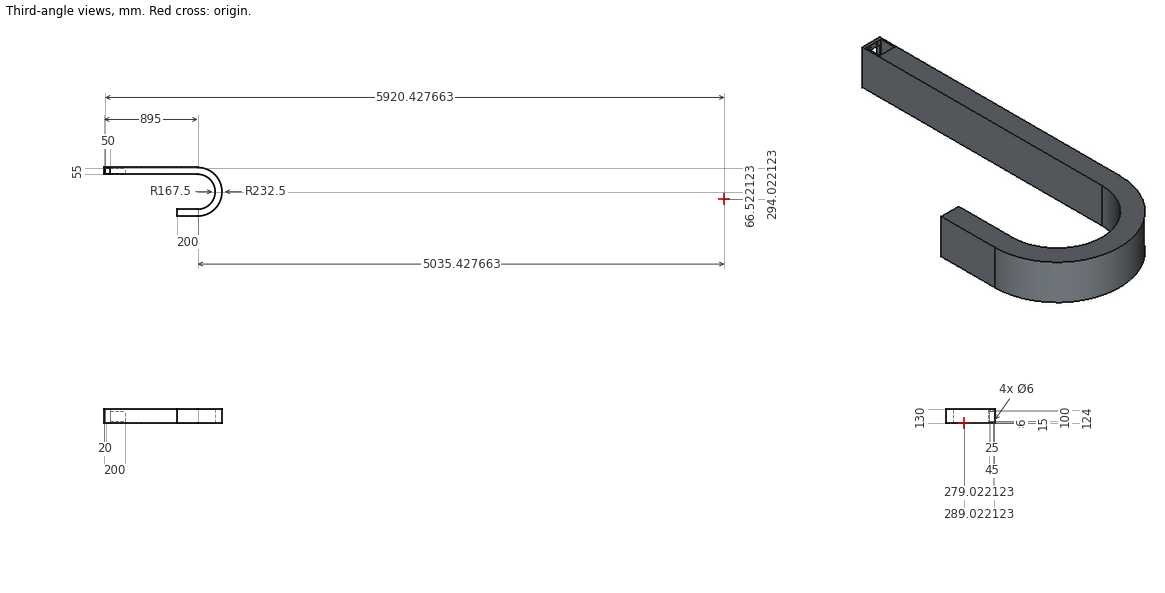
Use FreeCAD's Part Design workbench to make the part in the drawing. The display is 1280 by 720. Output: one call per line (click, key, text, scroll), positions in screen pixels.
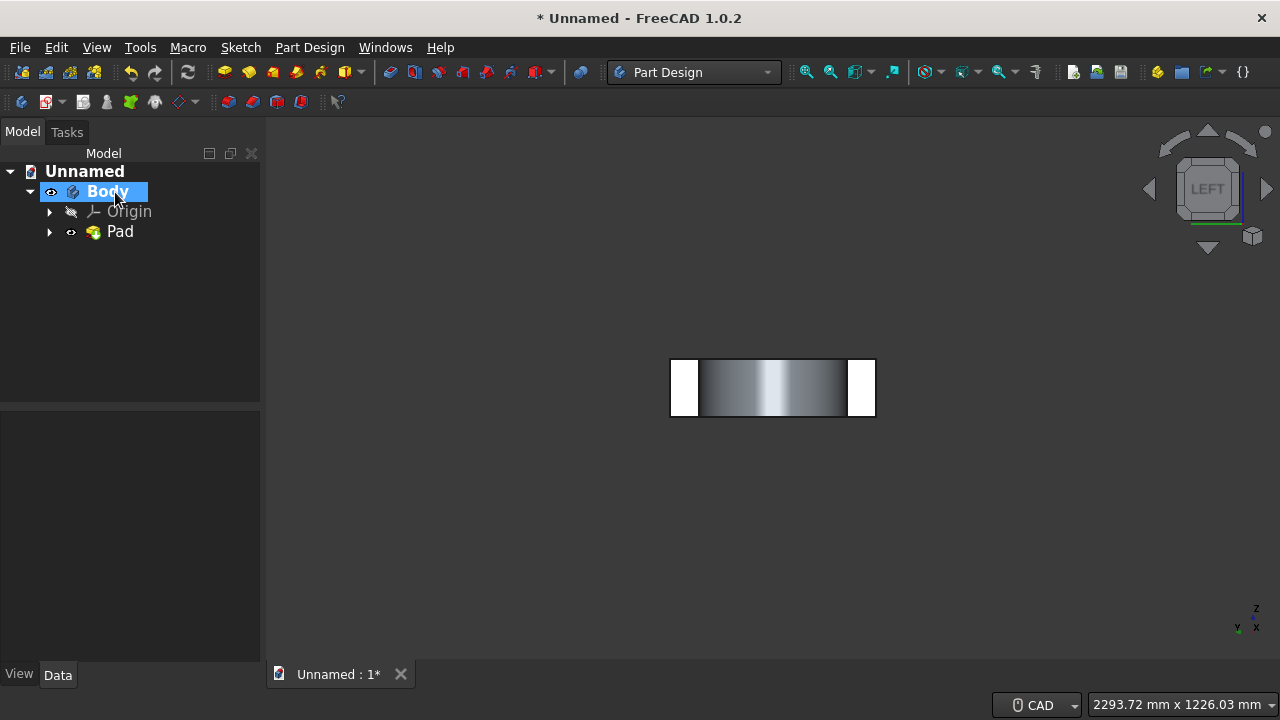
key(v)
key(f)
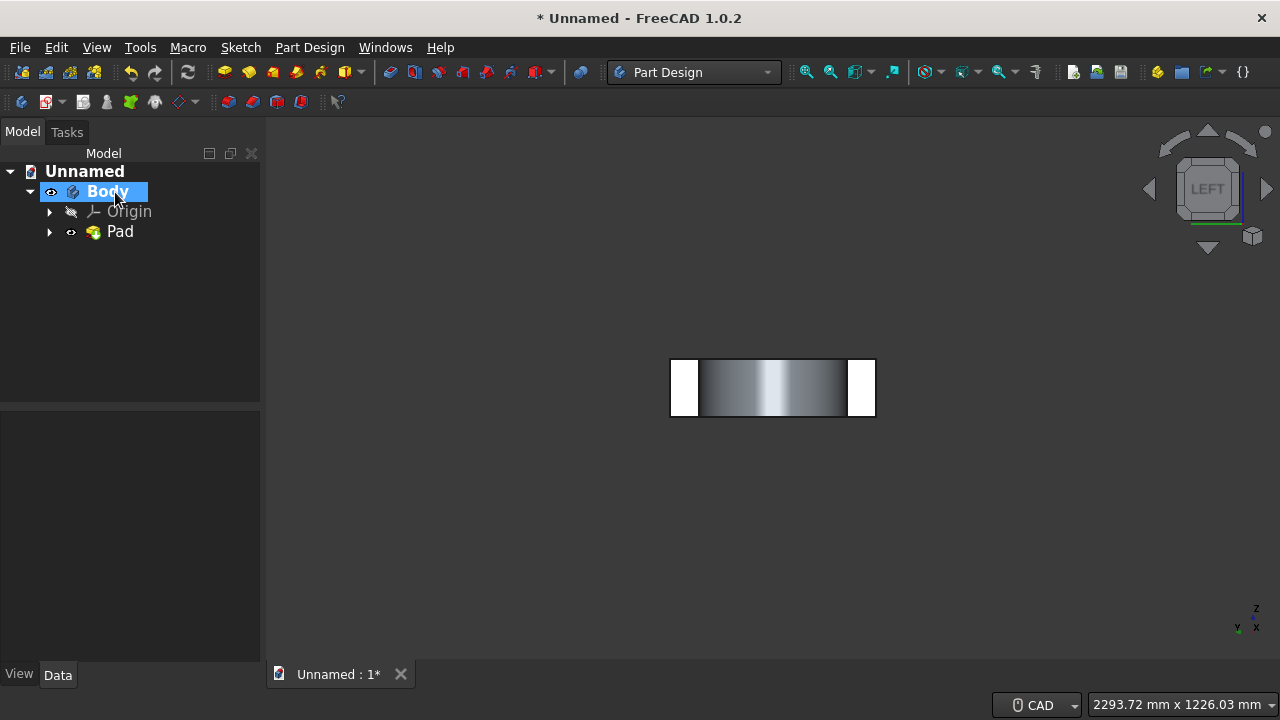
click(685, 379)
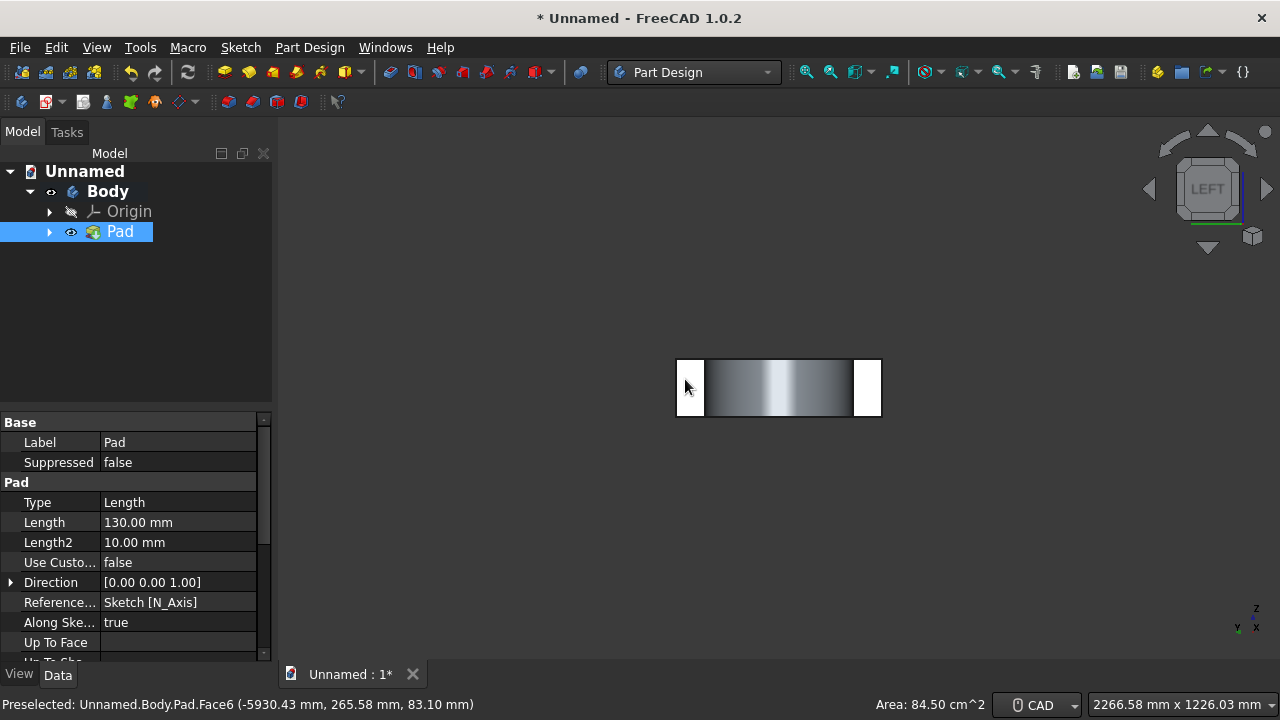
click(46, 102)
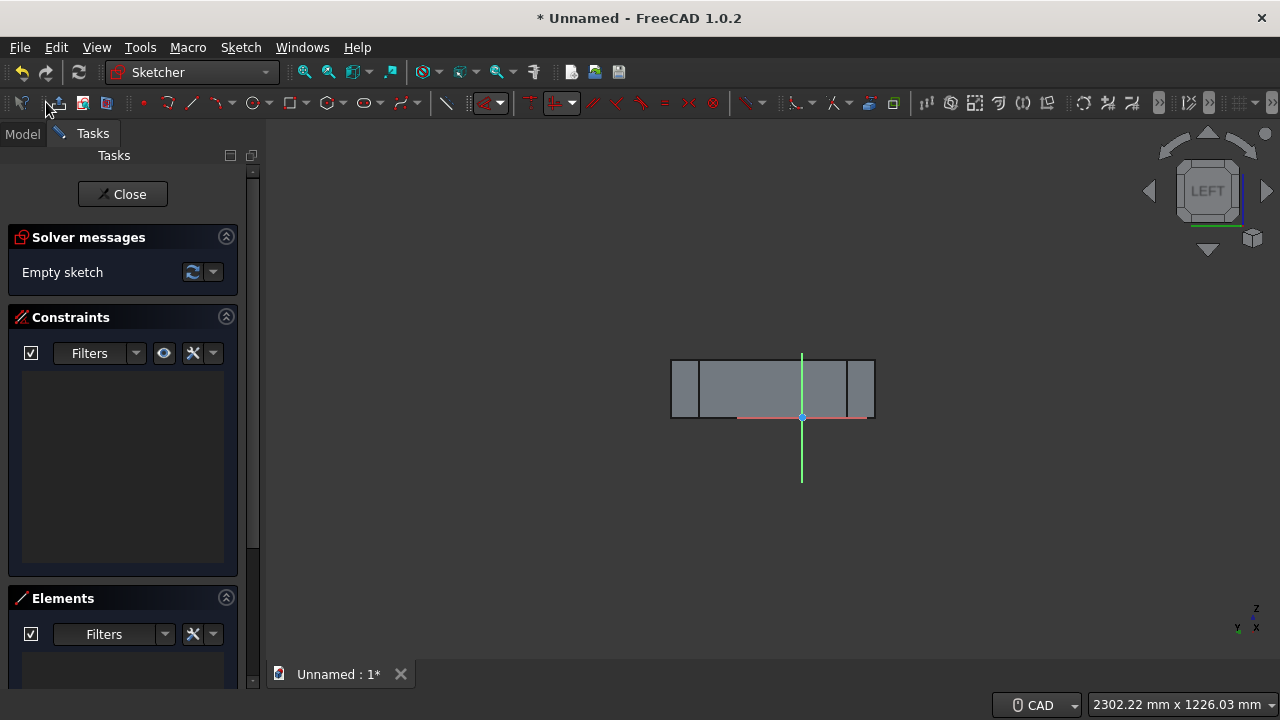
scroll(749, 390, up, 8)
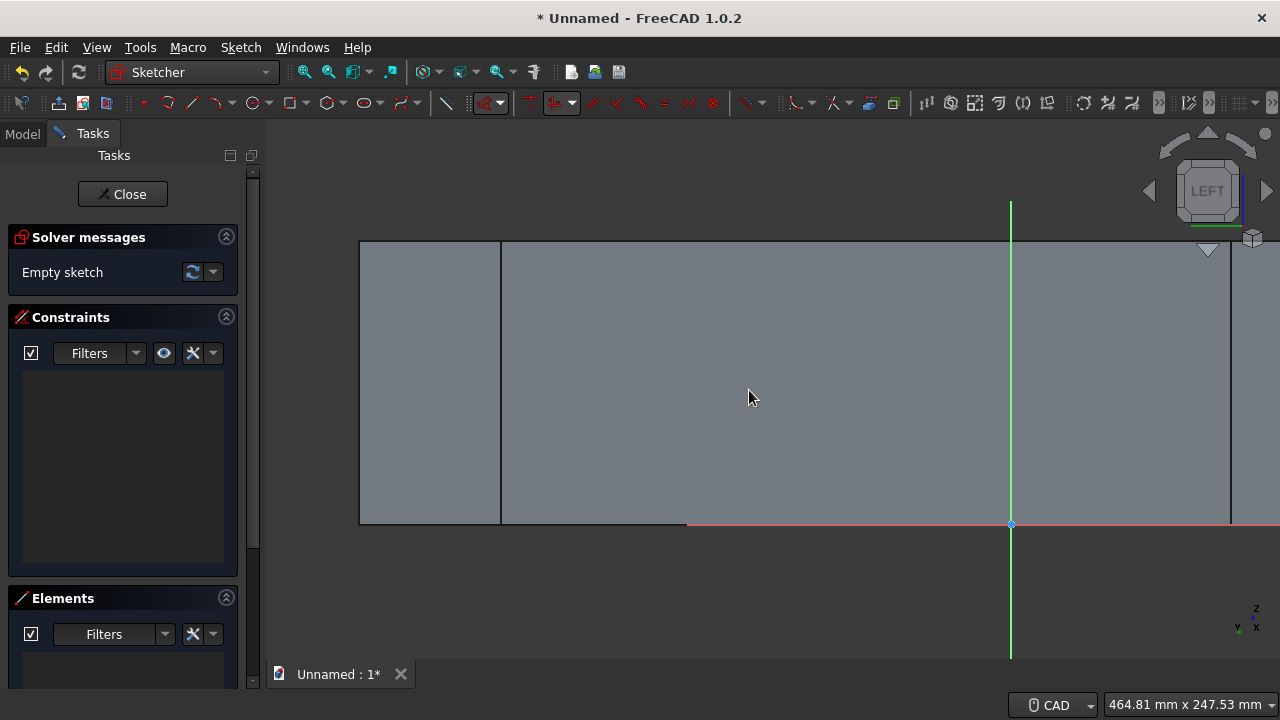
click(254, 104)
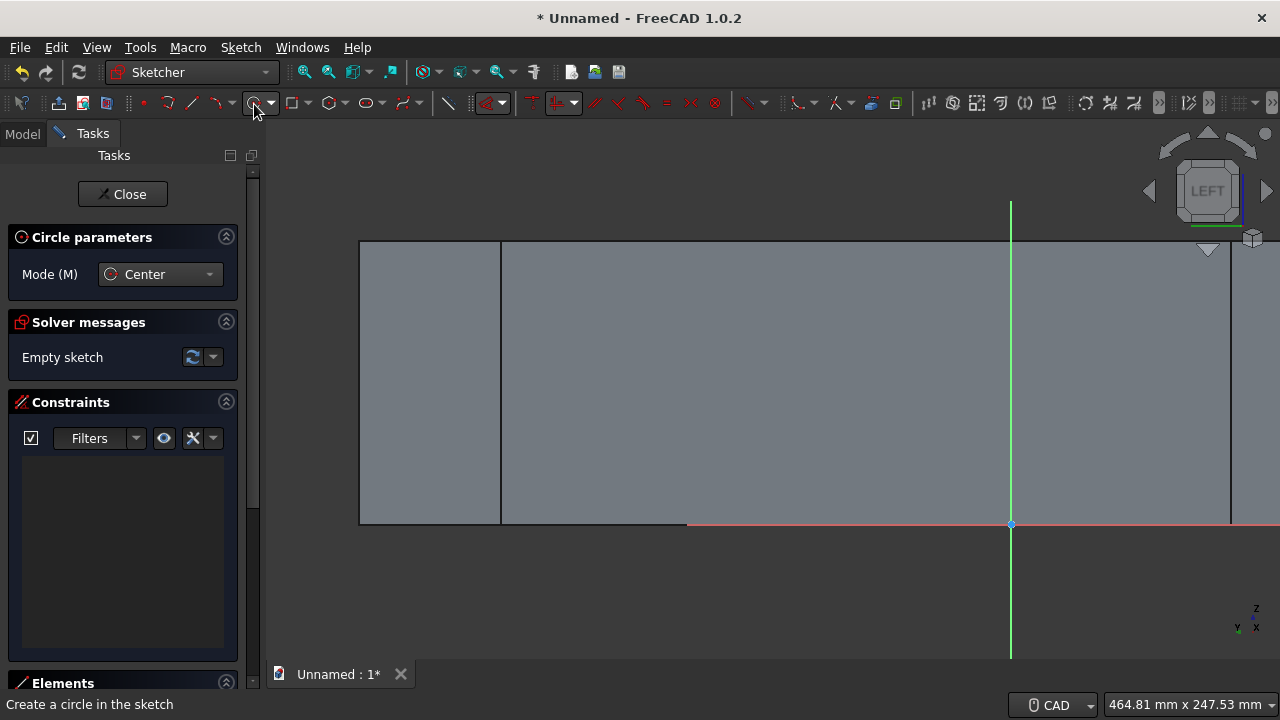
scroll(402, 512, up, 7)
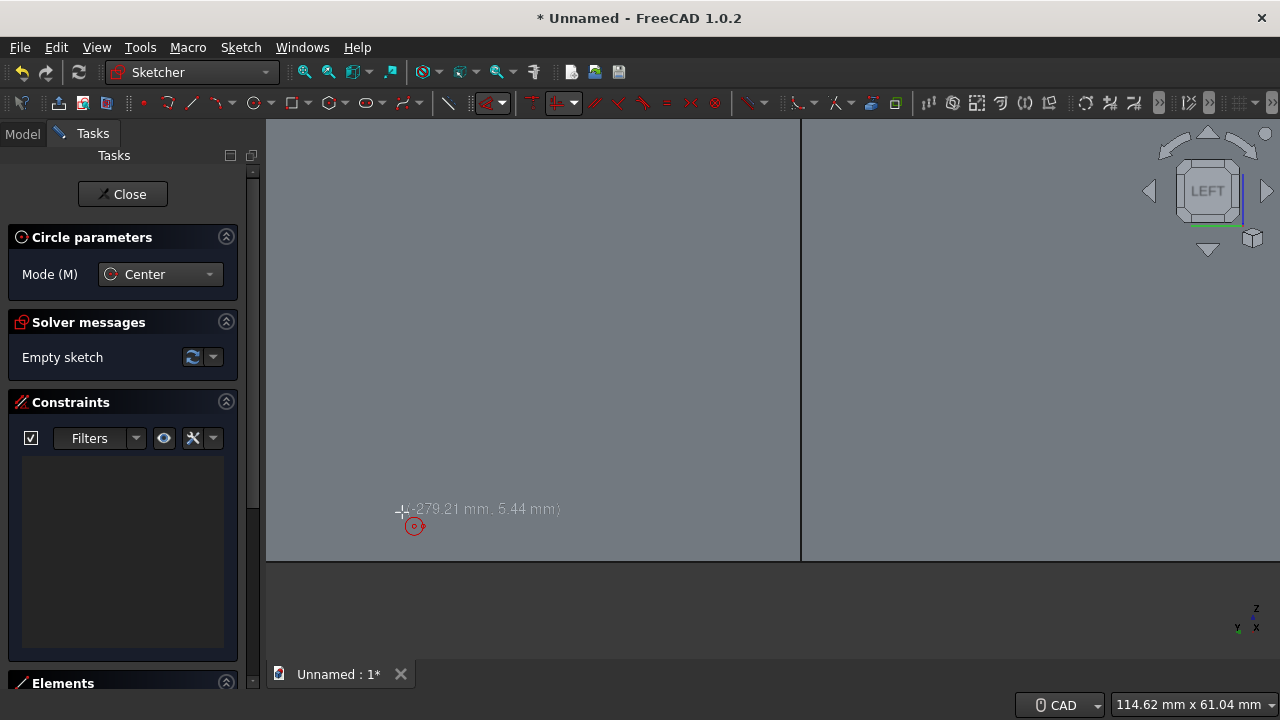
scroll(403, 516, down, 7)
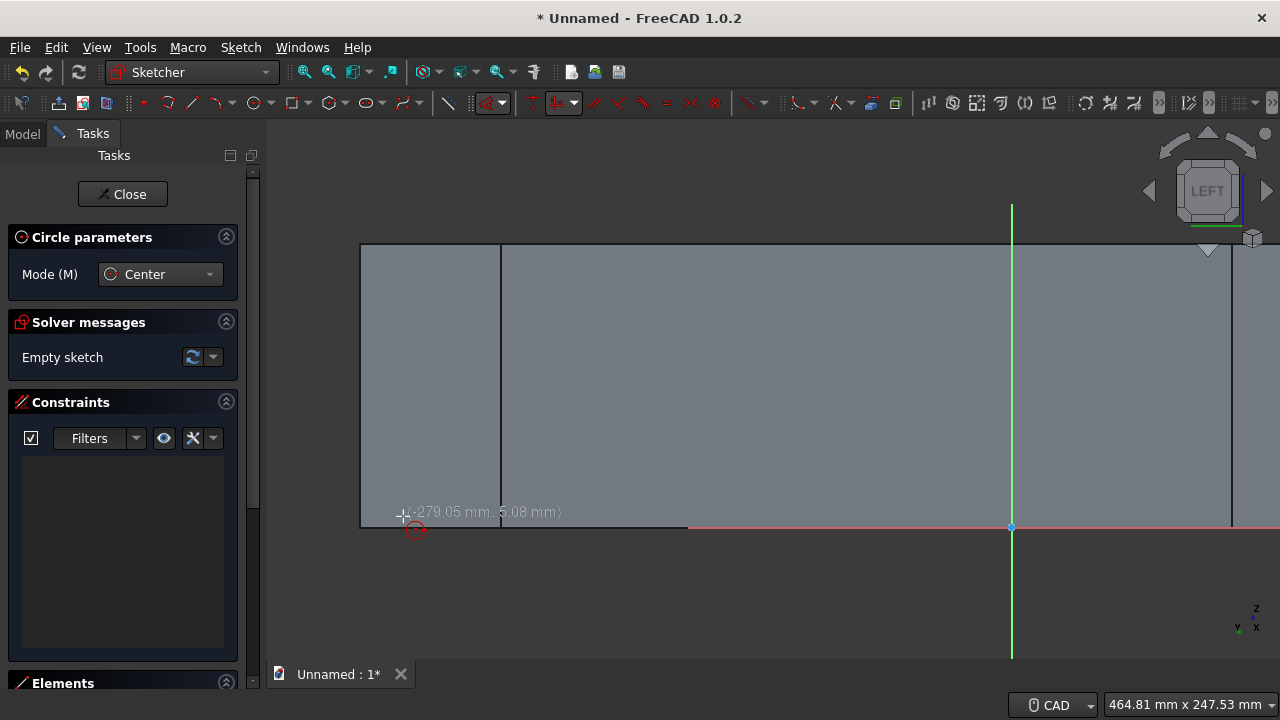
click(403, 515)
move(408, 510)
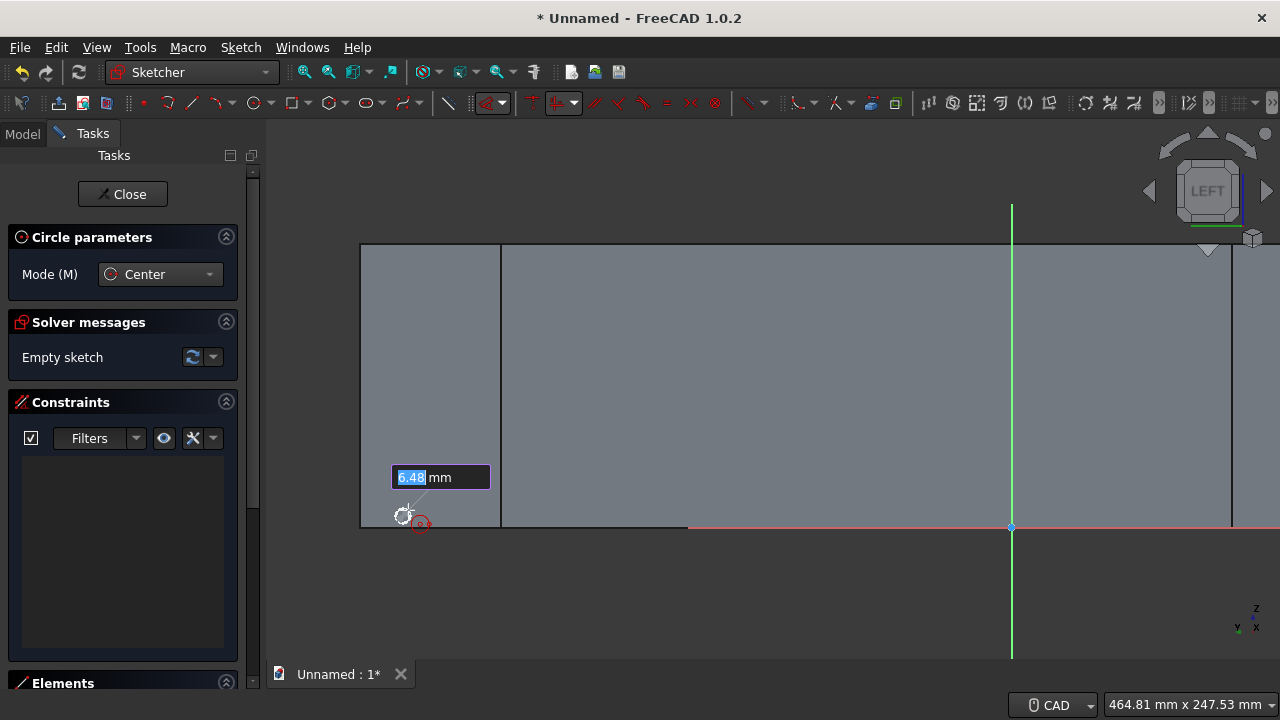
text(6)
key(Return)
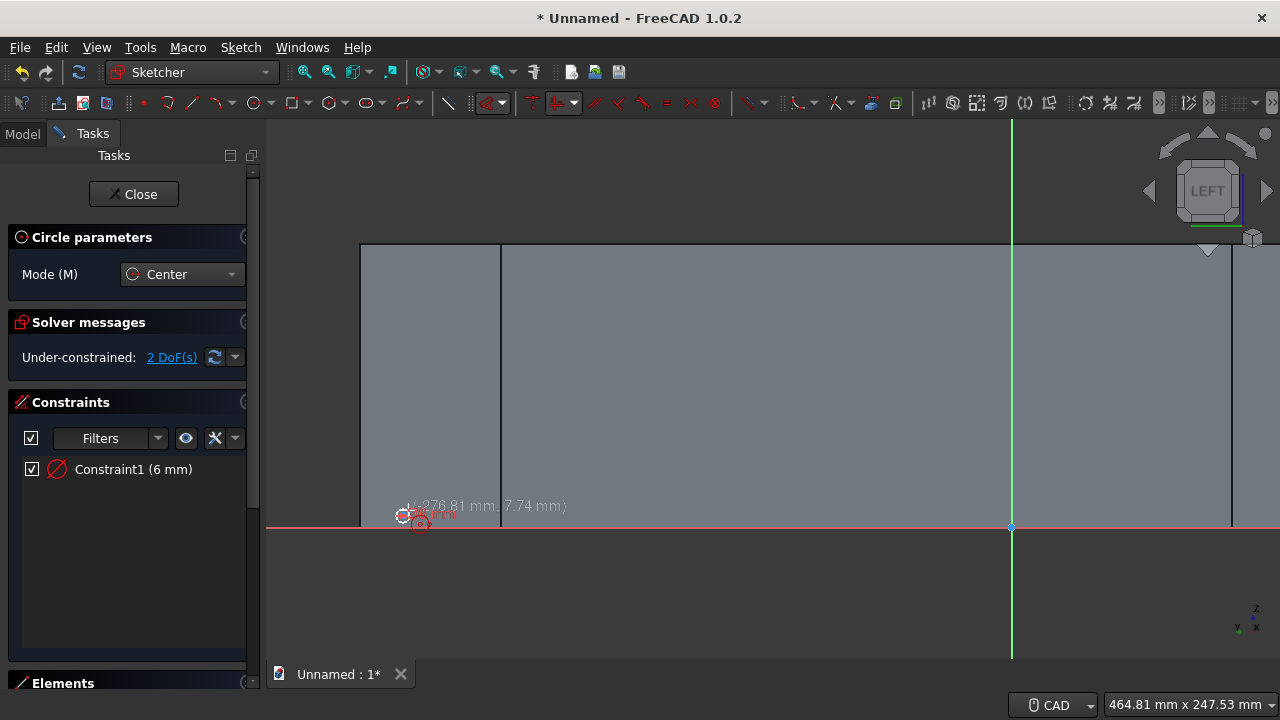
scroll(458, 515, up, 7)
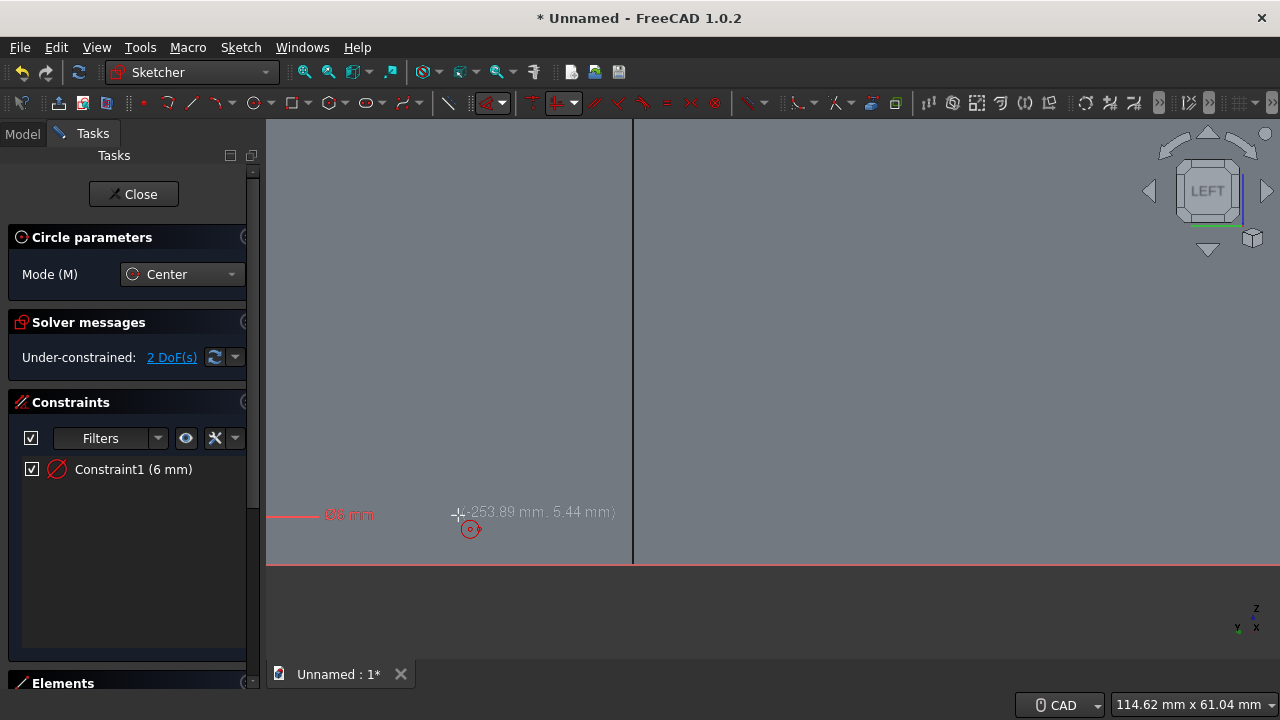
scroll(459, 515, down, 7)